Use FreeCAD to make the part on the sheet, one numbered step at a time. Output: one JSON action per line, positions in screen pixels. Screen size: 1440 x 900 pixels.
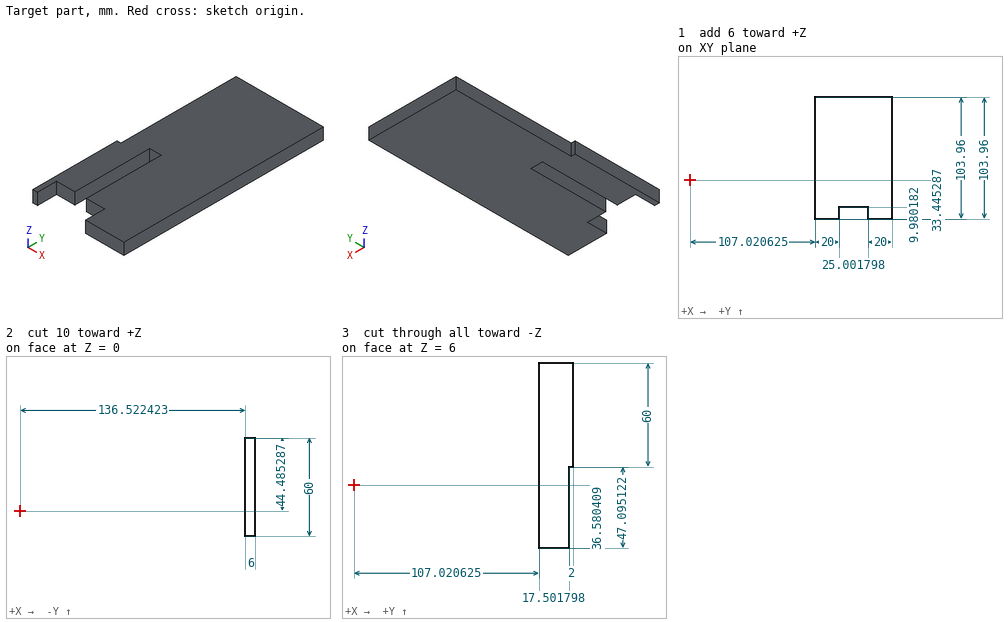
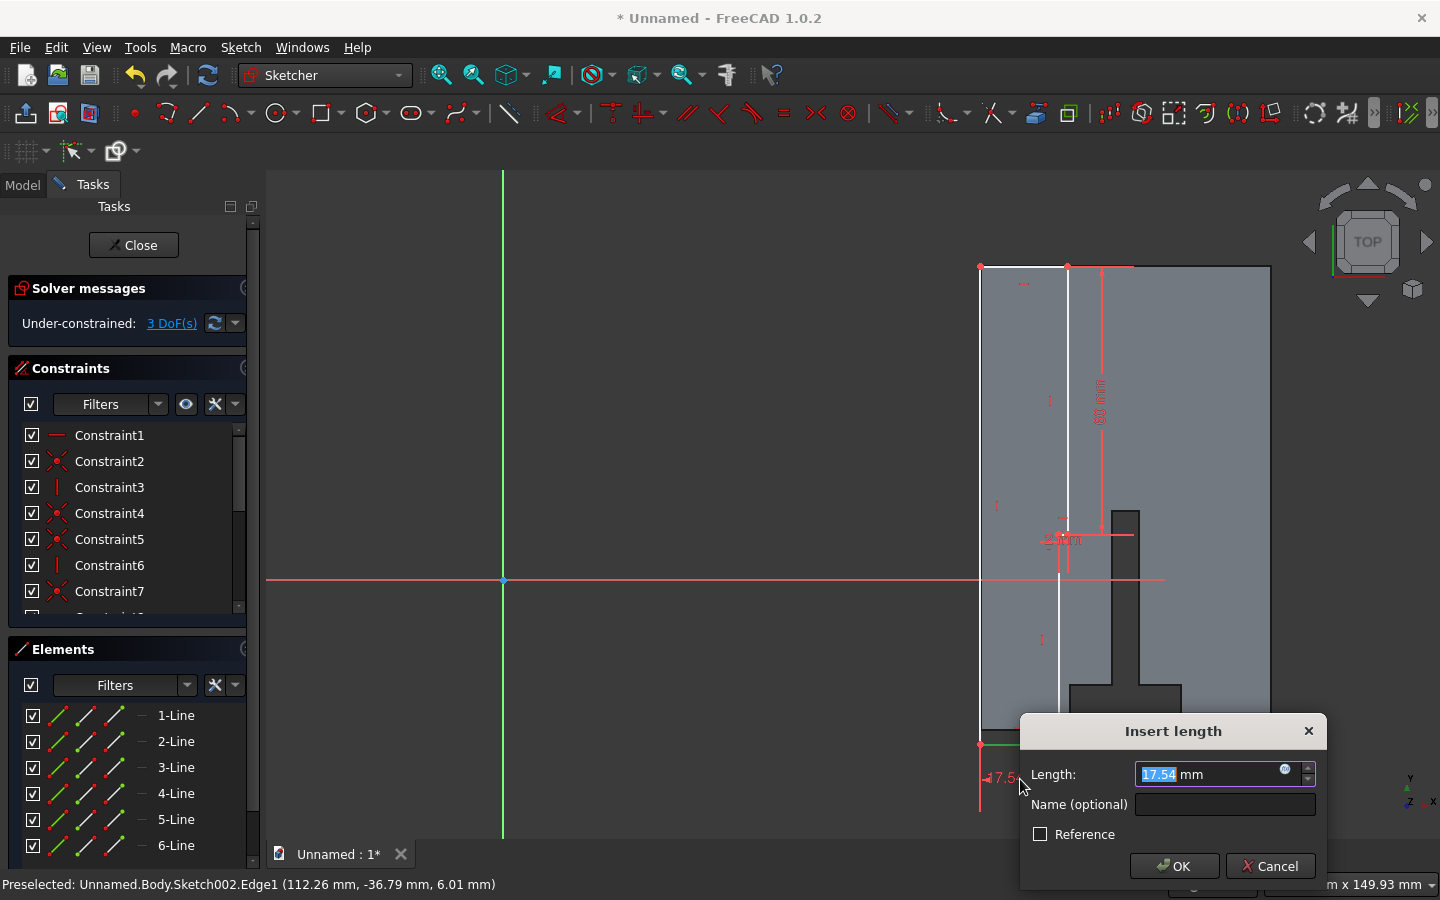
{"action": "type", "text": "17.501798"}
{"action": "key", "text": "Return"}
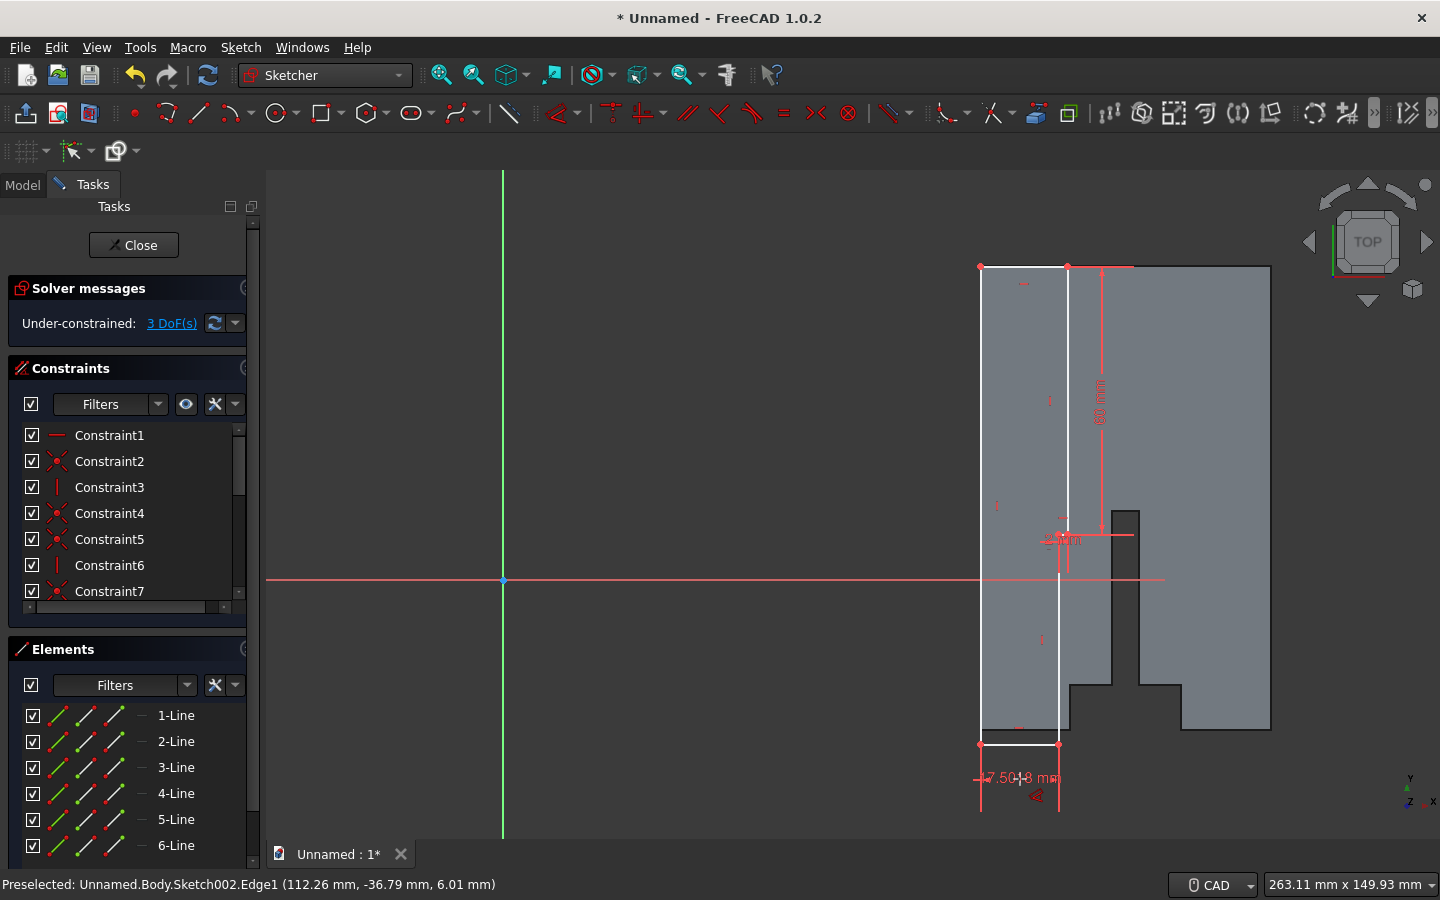
{"action": "left_click", "coordinate": [1059, 682]}
{"action": "left_click", "coordinate": [1093, 640]}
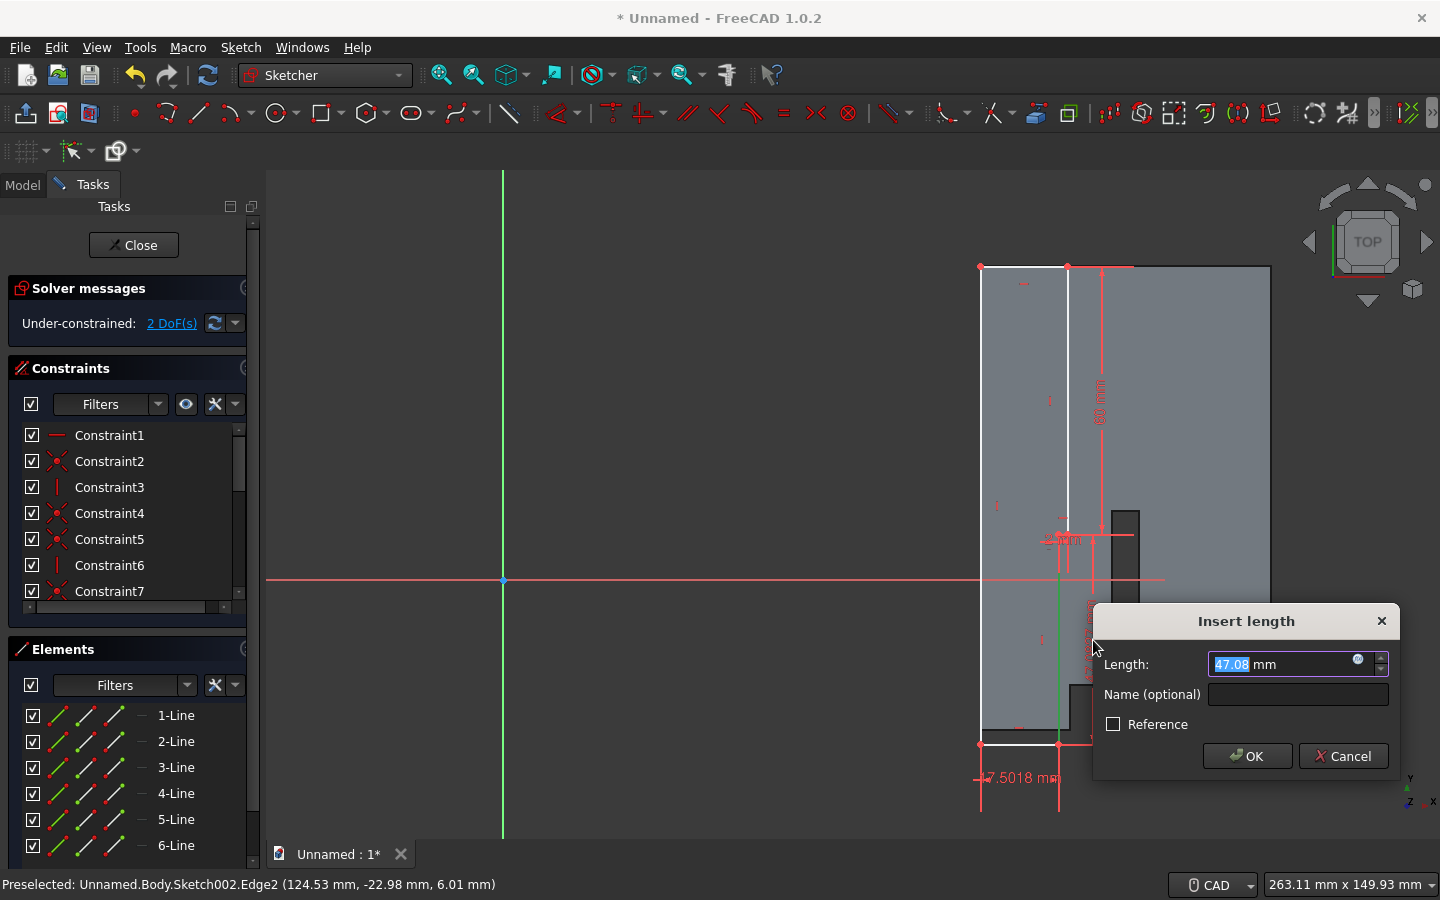
{"action": "type", "text": "47.095122"}
{"action": "key", "text": "Return"}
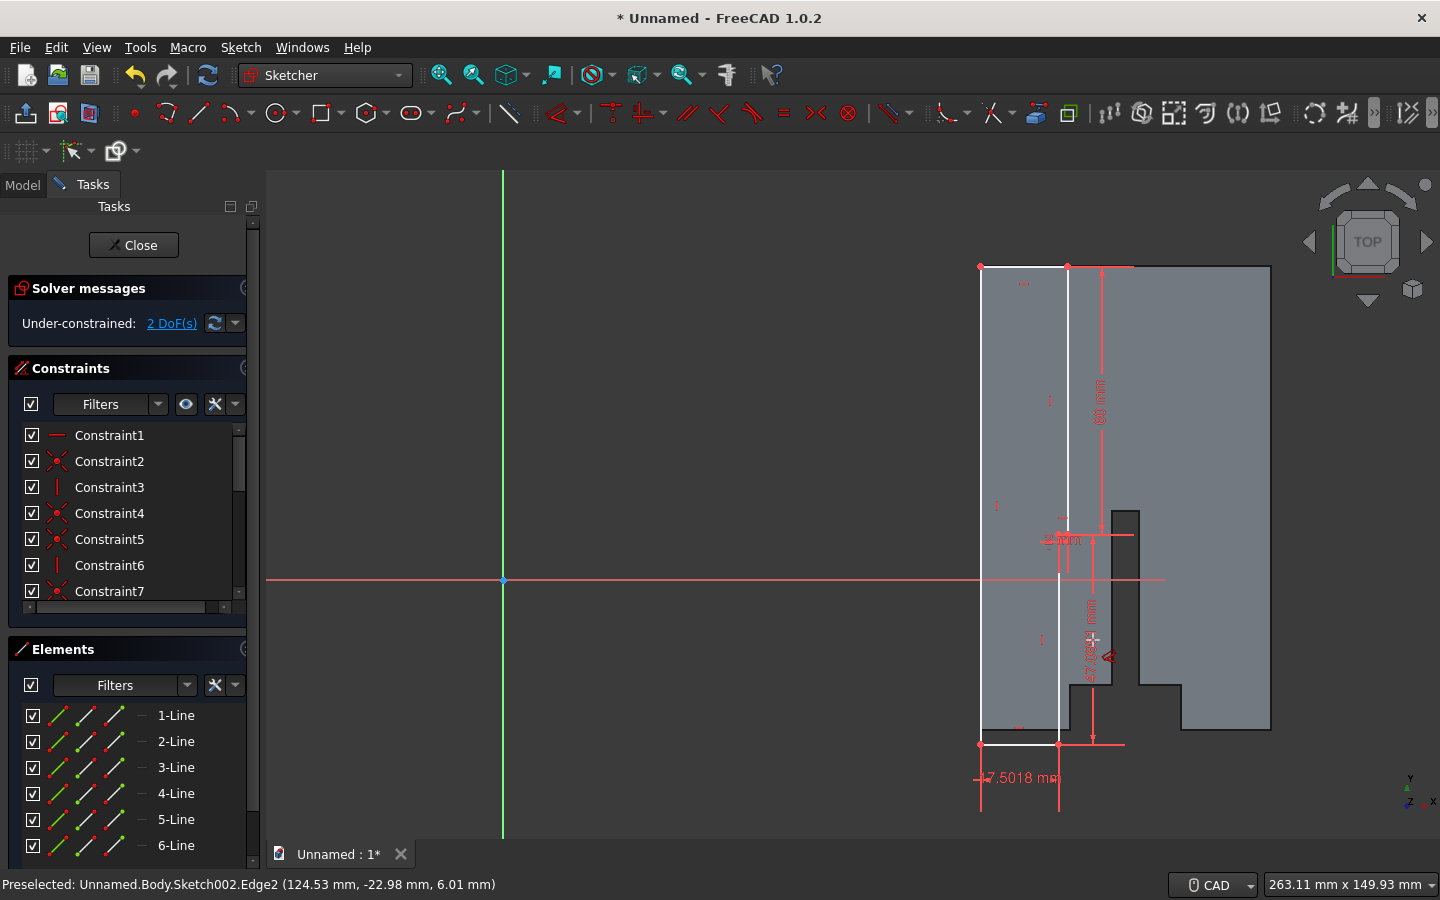
{"action": "left_click", "coordinate": [981, 745]}
{"action": "left_click", "coordinate": [469, 663]}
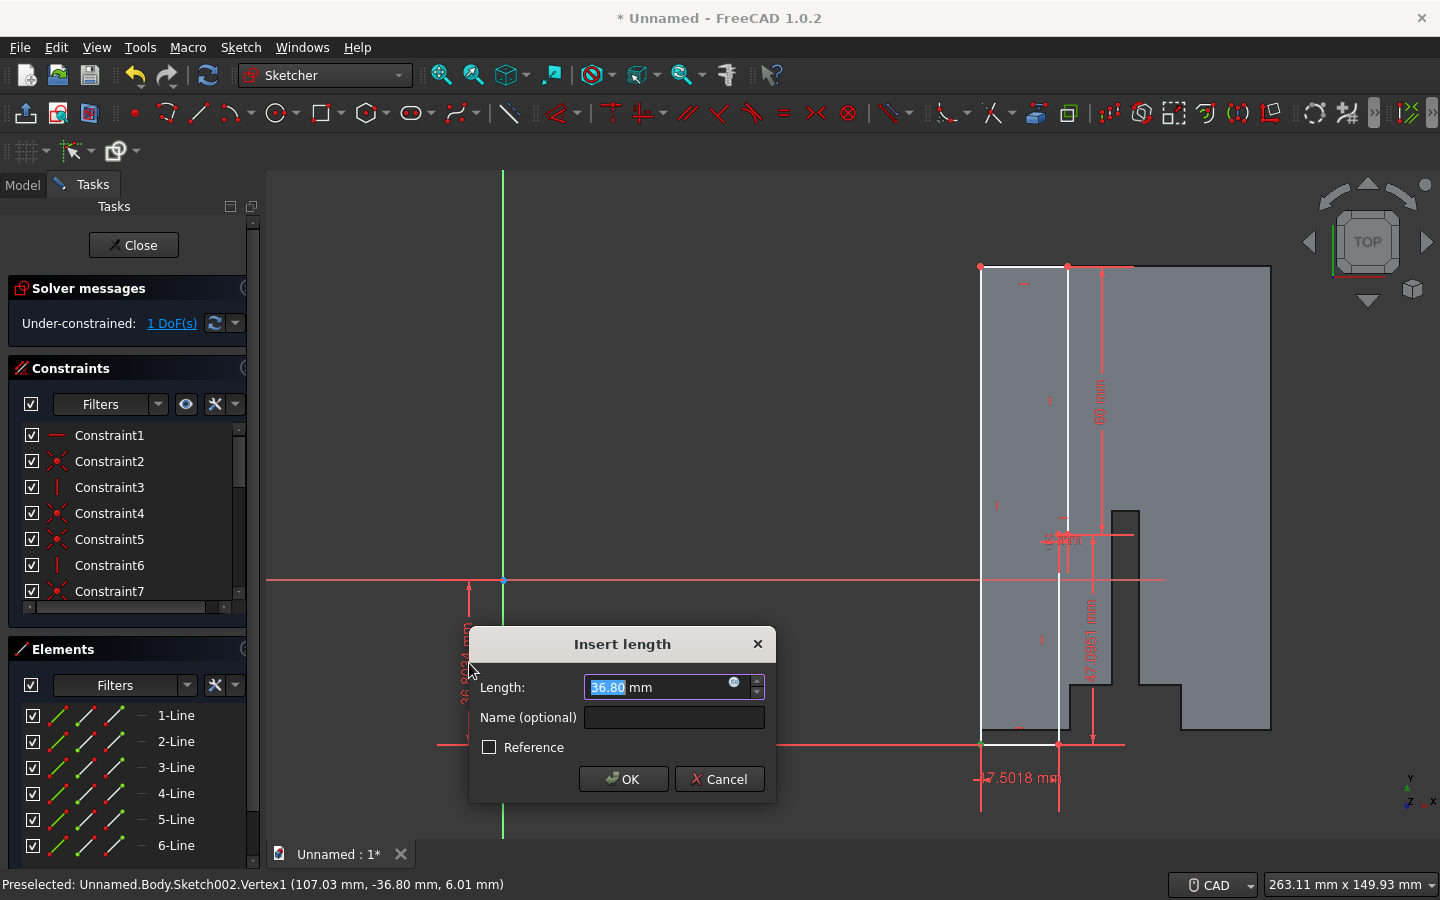
{"action": "type", "text": "36.580409"}
{"action": "key", "text": "Return"}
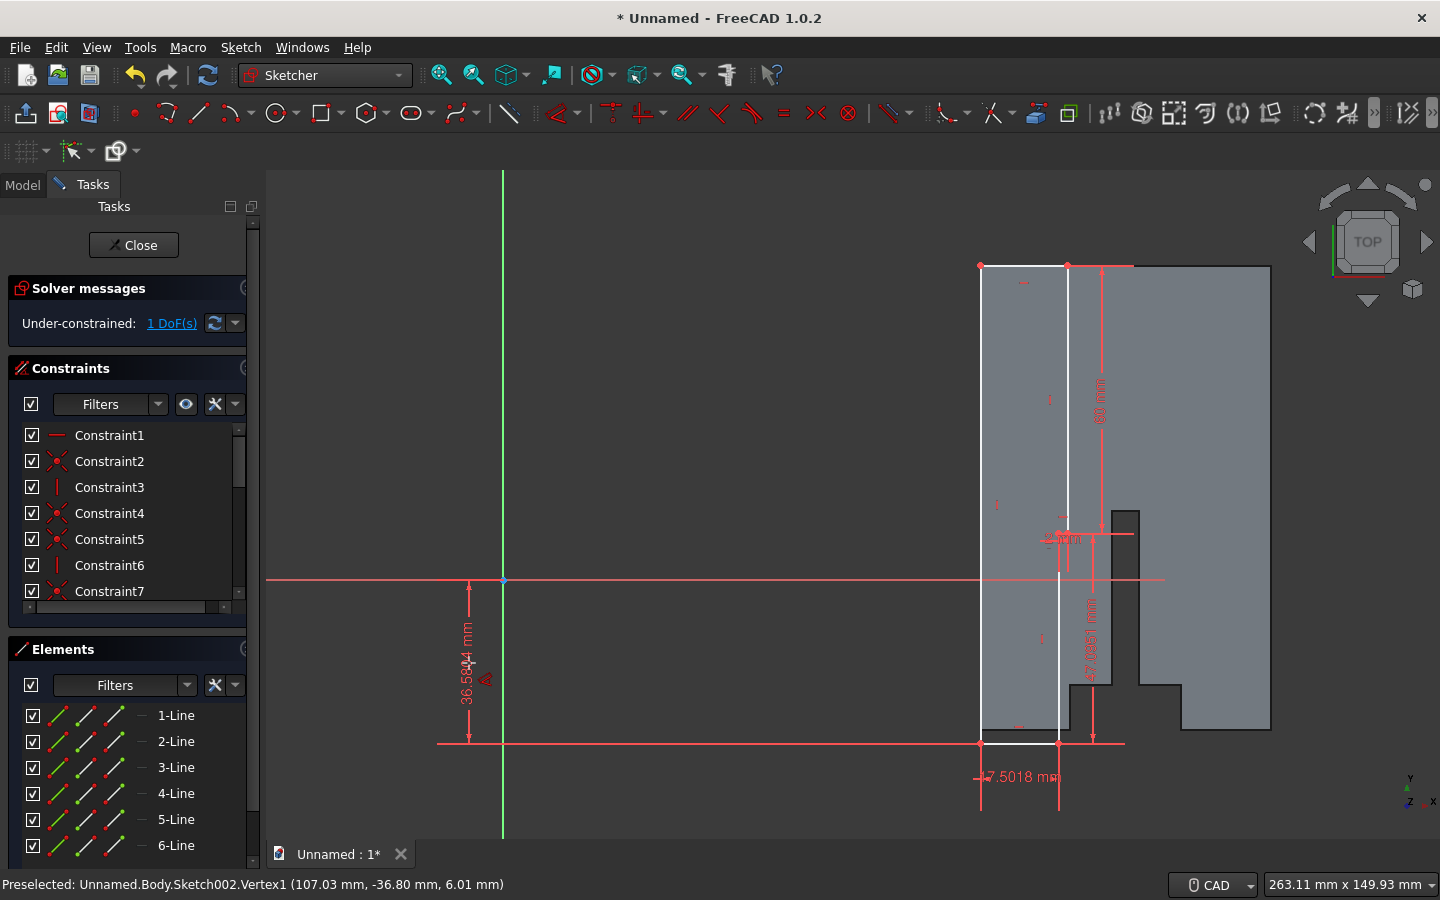
{"action": "left_click", "coordinate": [981, 744]}
{"action": "left_click", "coordinate": [742, 778]}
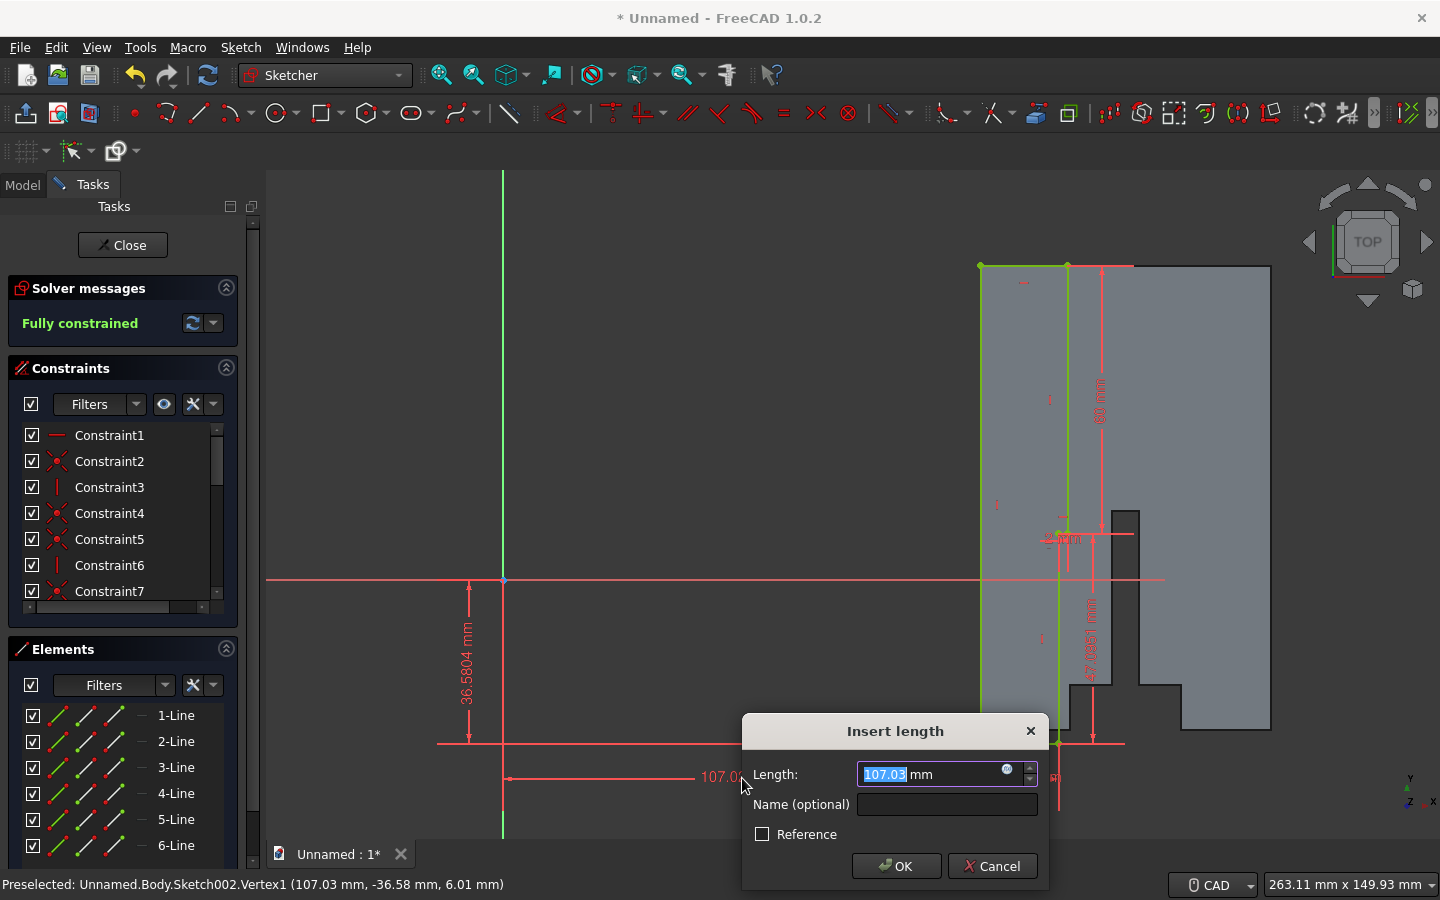
{"action": "type", "text": "107.020625"}
{"action": "key", "text": "Return"}
{"action": "key", "text": "Escape"}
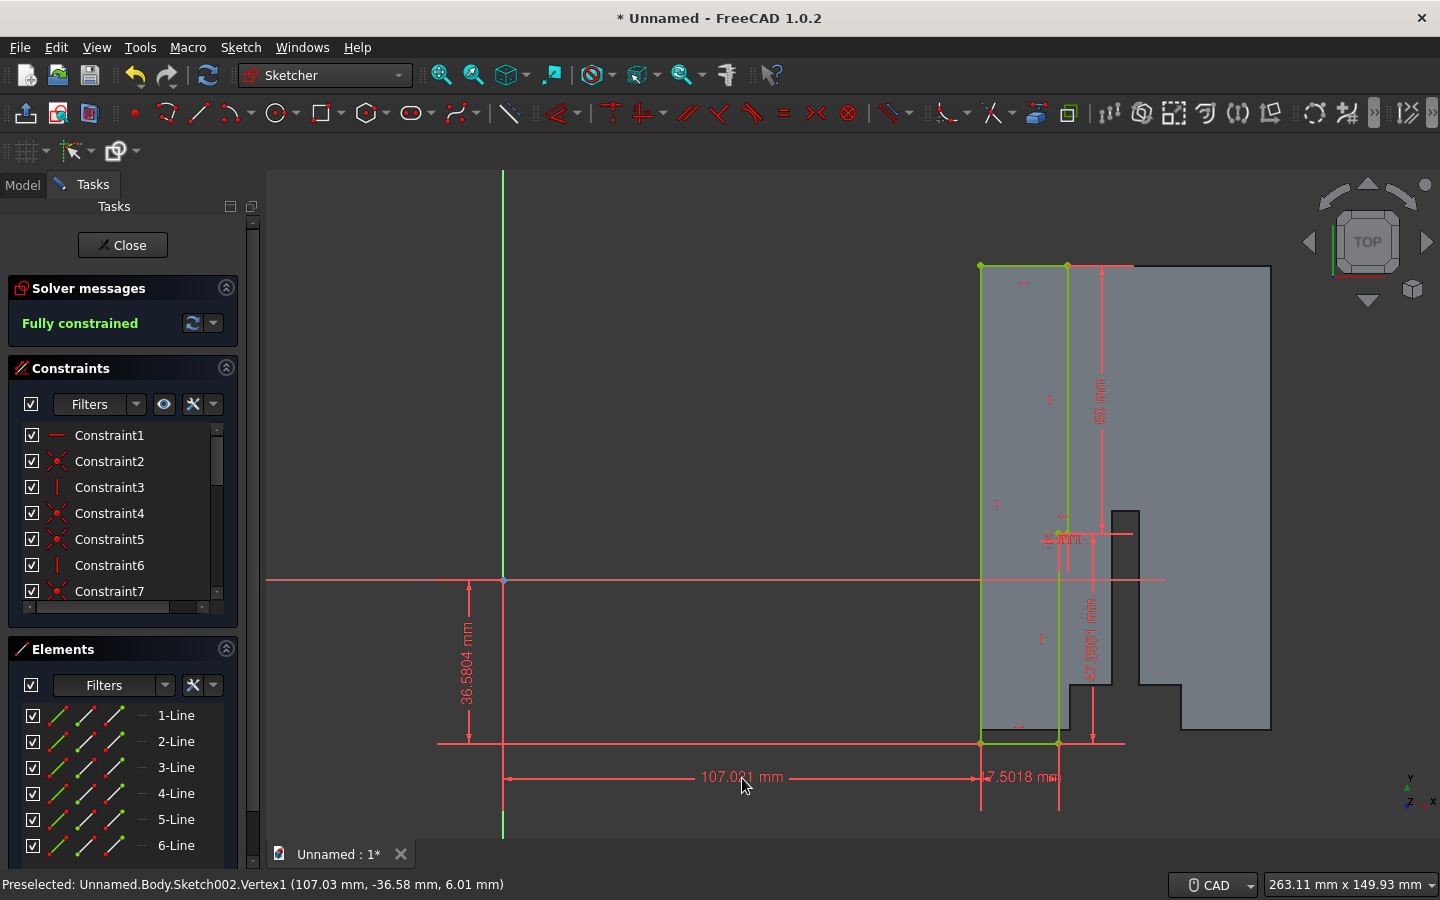
{"action": "left_click", "coordinate": [123, 245]}